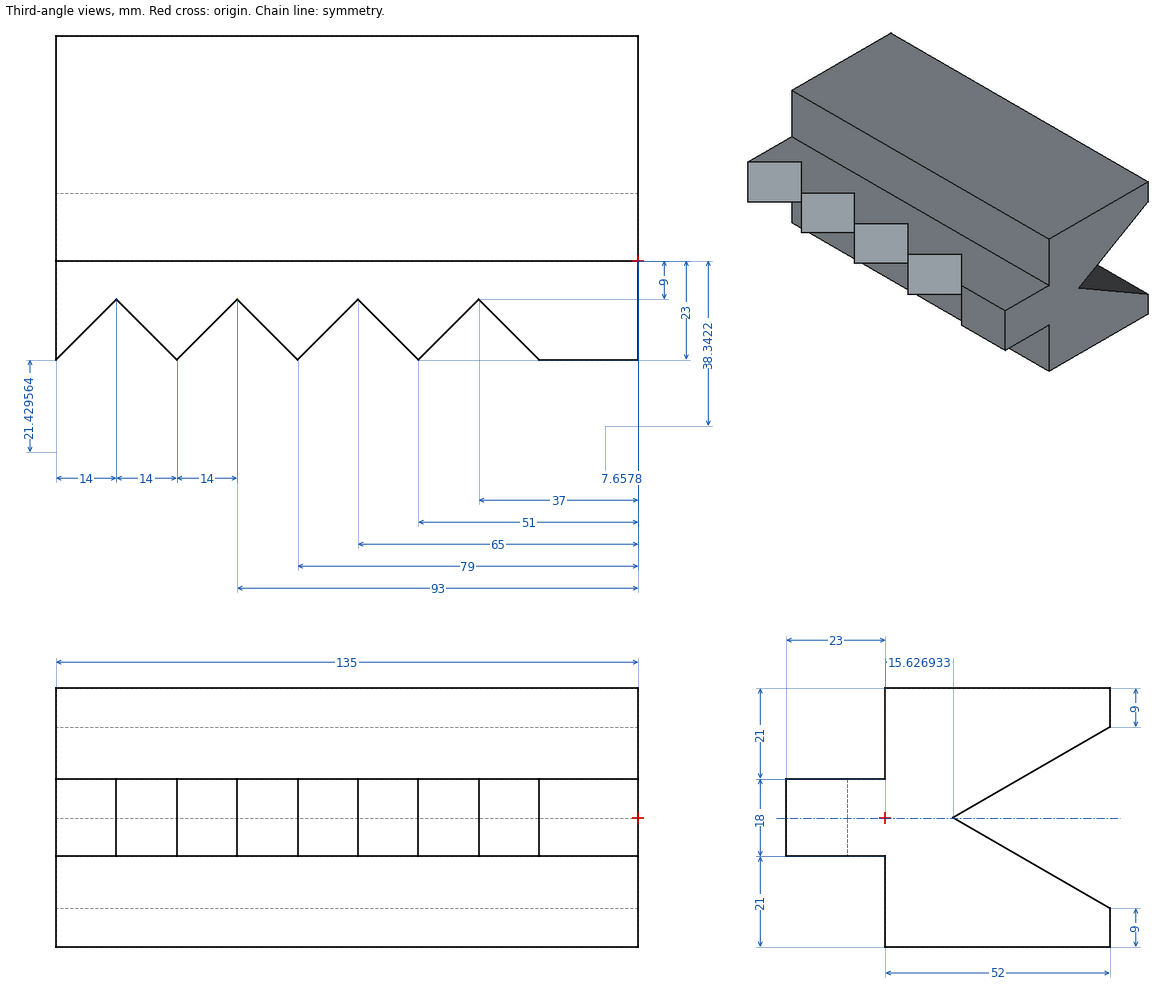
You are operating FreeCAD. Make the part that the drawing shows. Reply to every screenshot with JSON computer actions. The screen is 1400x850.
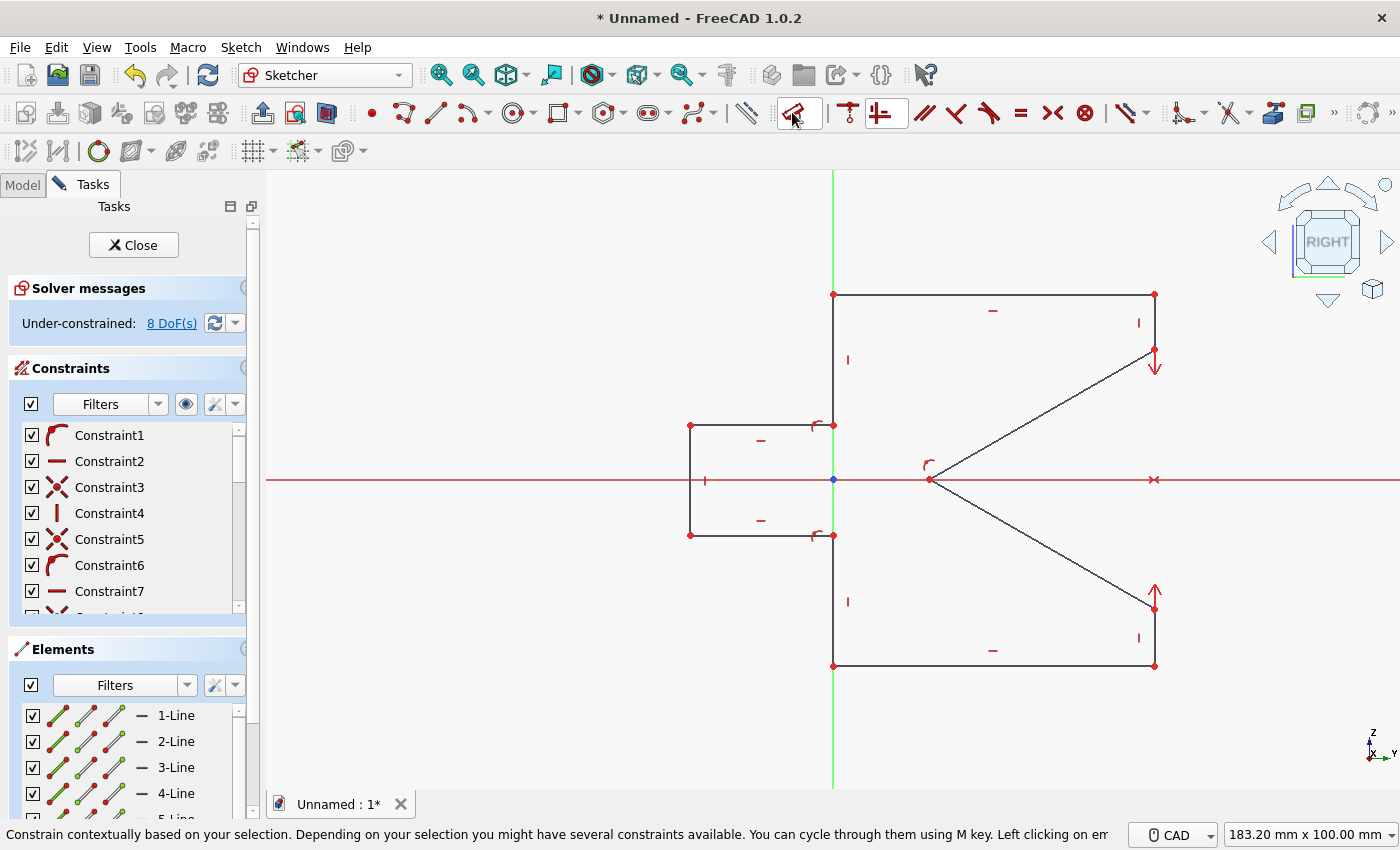
{"action": "left_click", "coordinate": [1155, 649]}
{"action": "left_click", "coordinate": [1189, 638]}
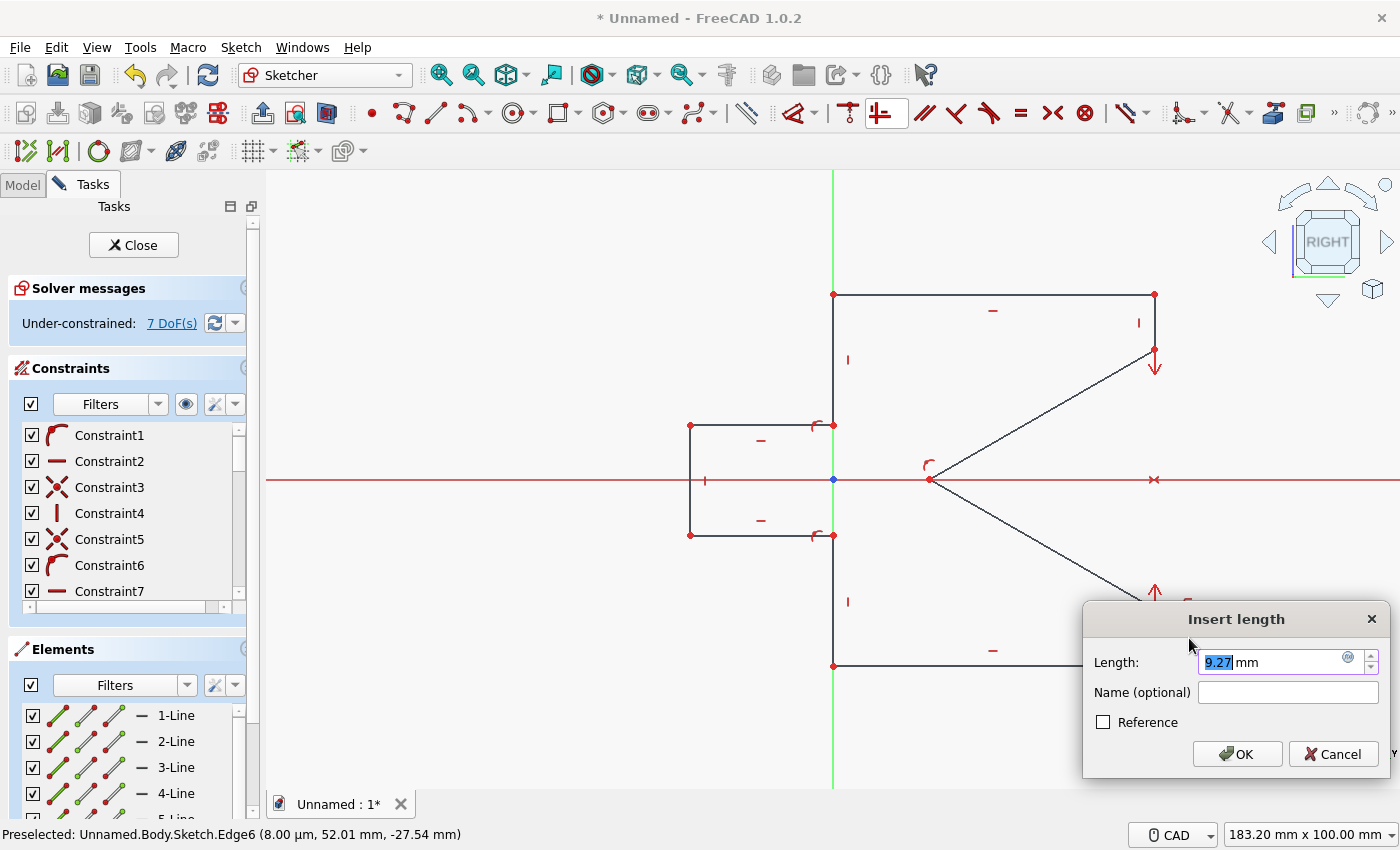
{"action": "type", "text": "9"}
{"action": "key", "text": "Return"}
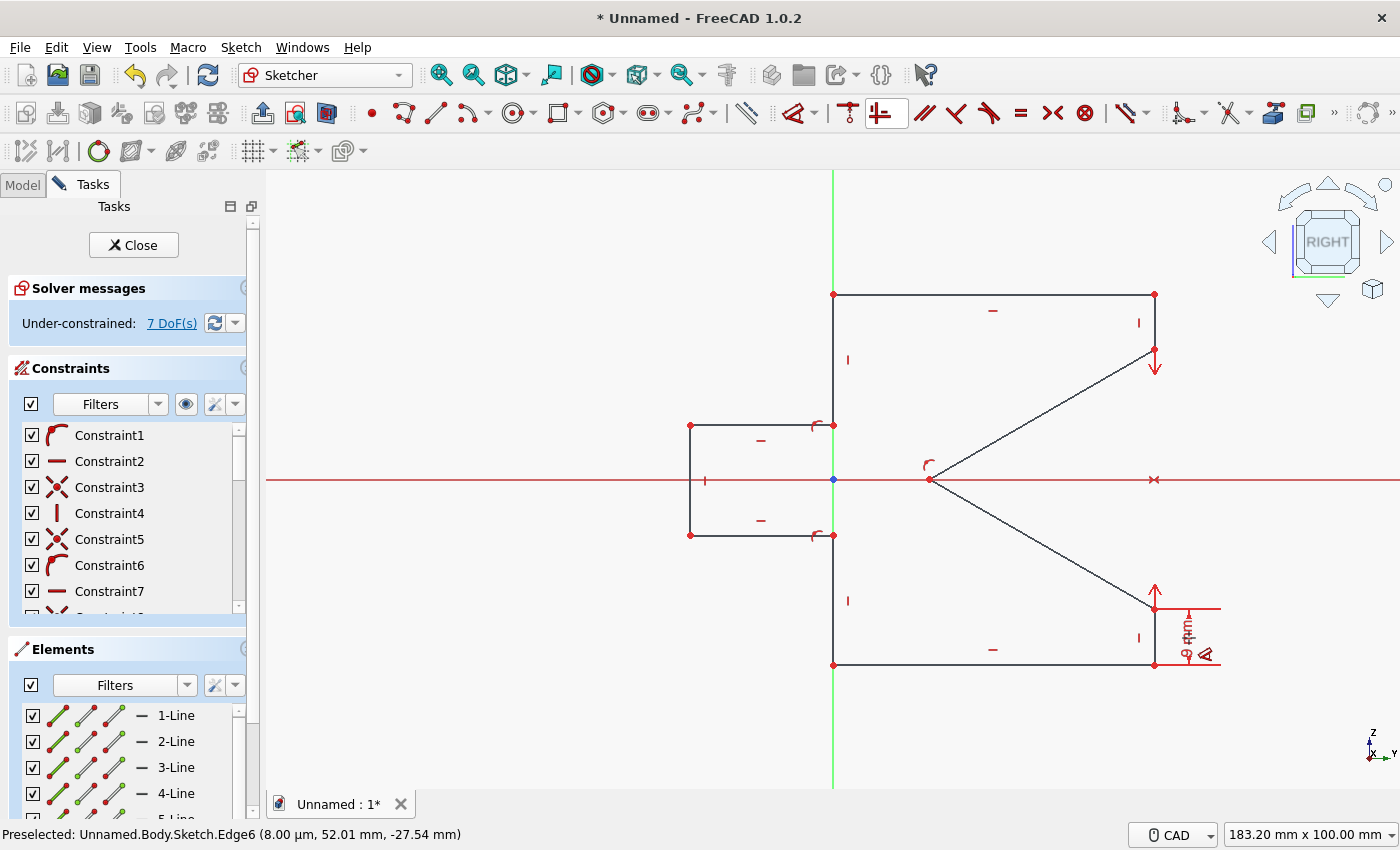
{"action": "left_click", "coordinate": [1155, 333]}
{"action": "left_click", "coordinate": [1189, 322]}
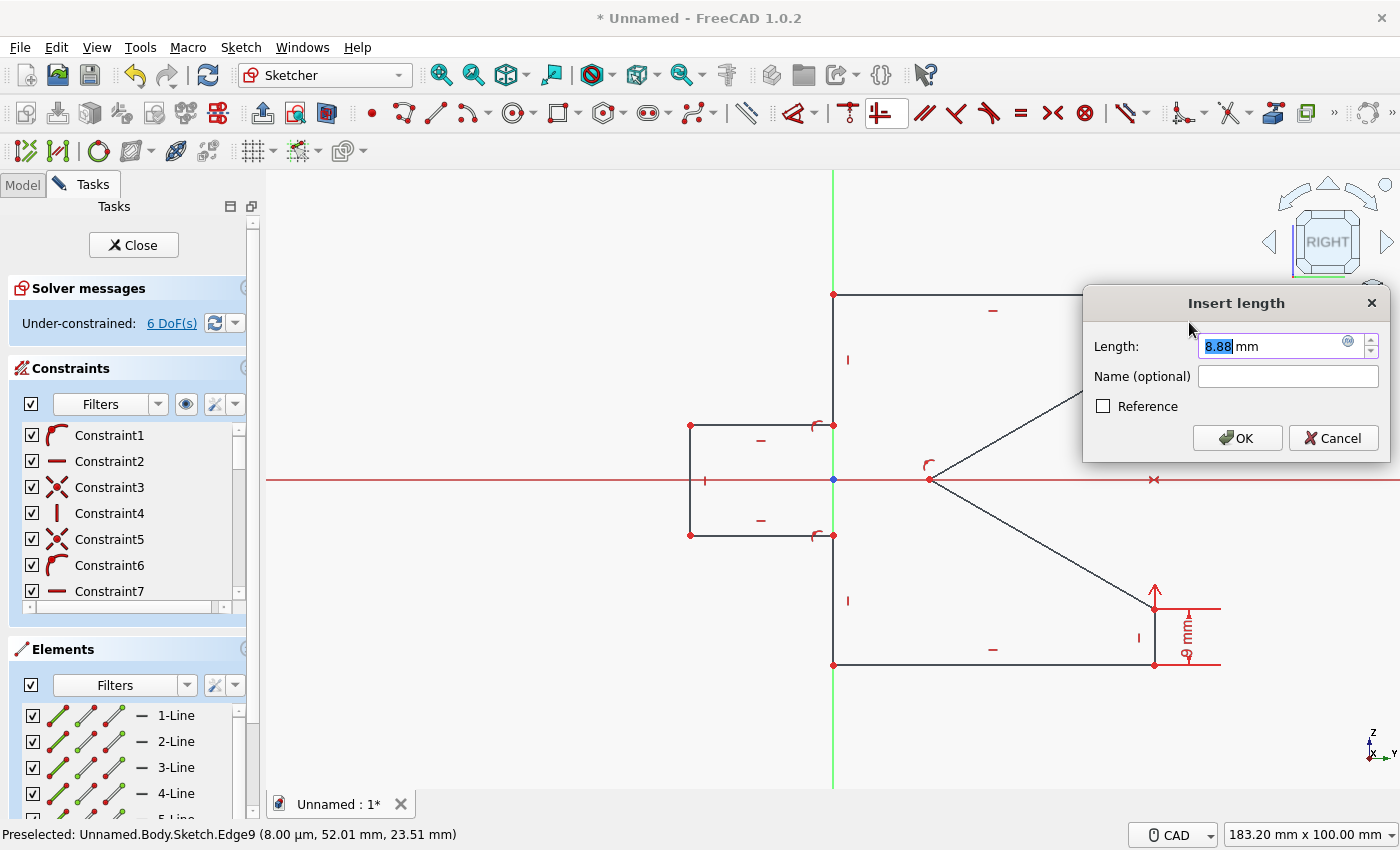
{"action": "type", "text": "9"}
{"action": "key", "text": "Return"}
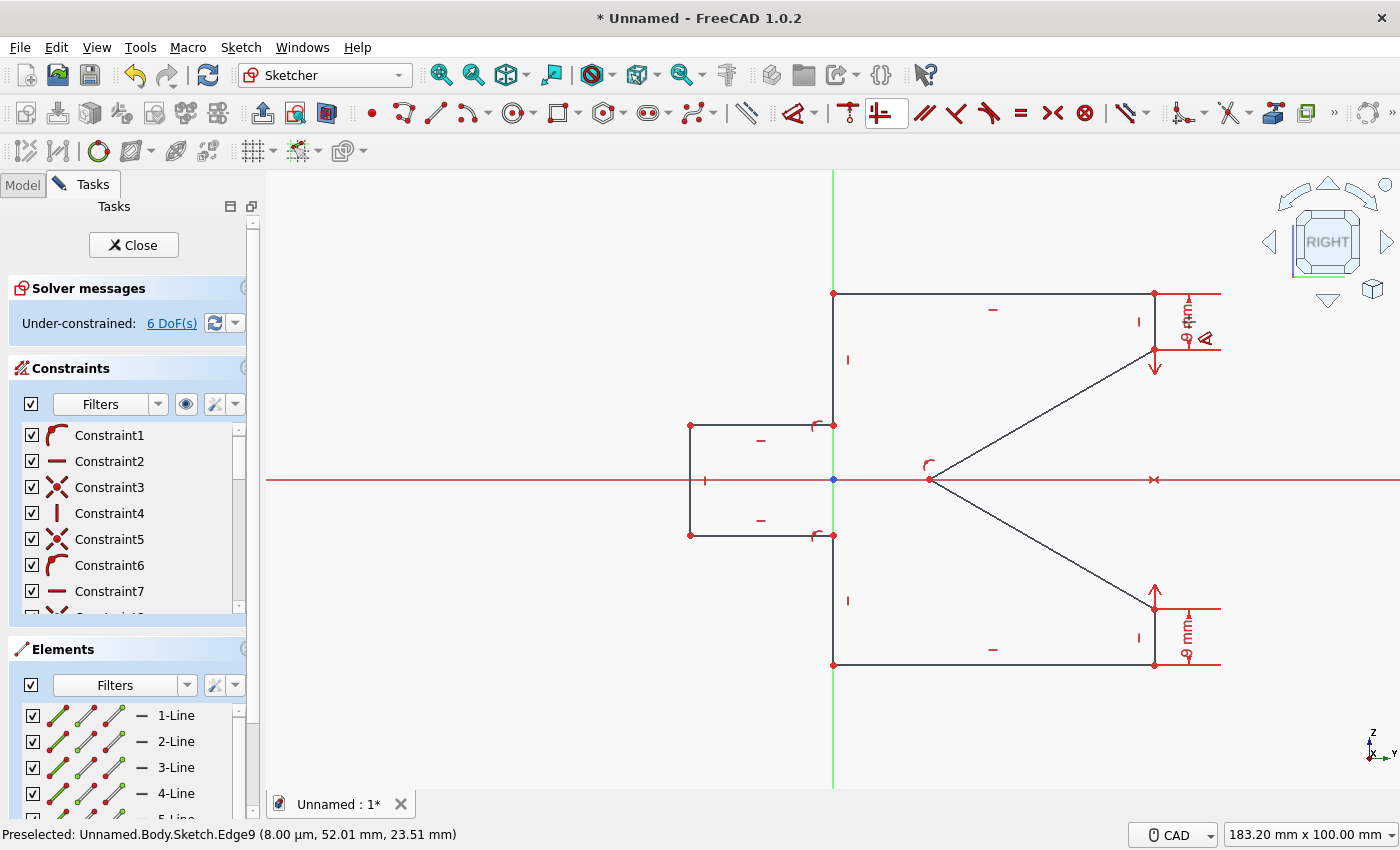
{"action": "left_click", "coordinate": [790, 425]}
{"action": "left_click", "coordinate": [762, 391]}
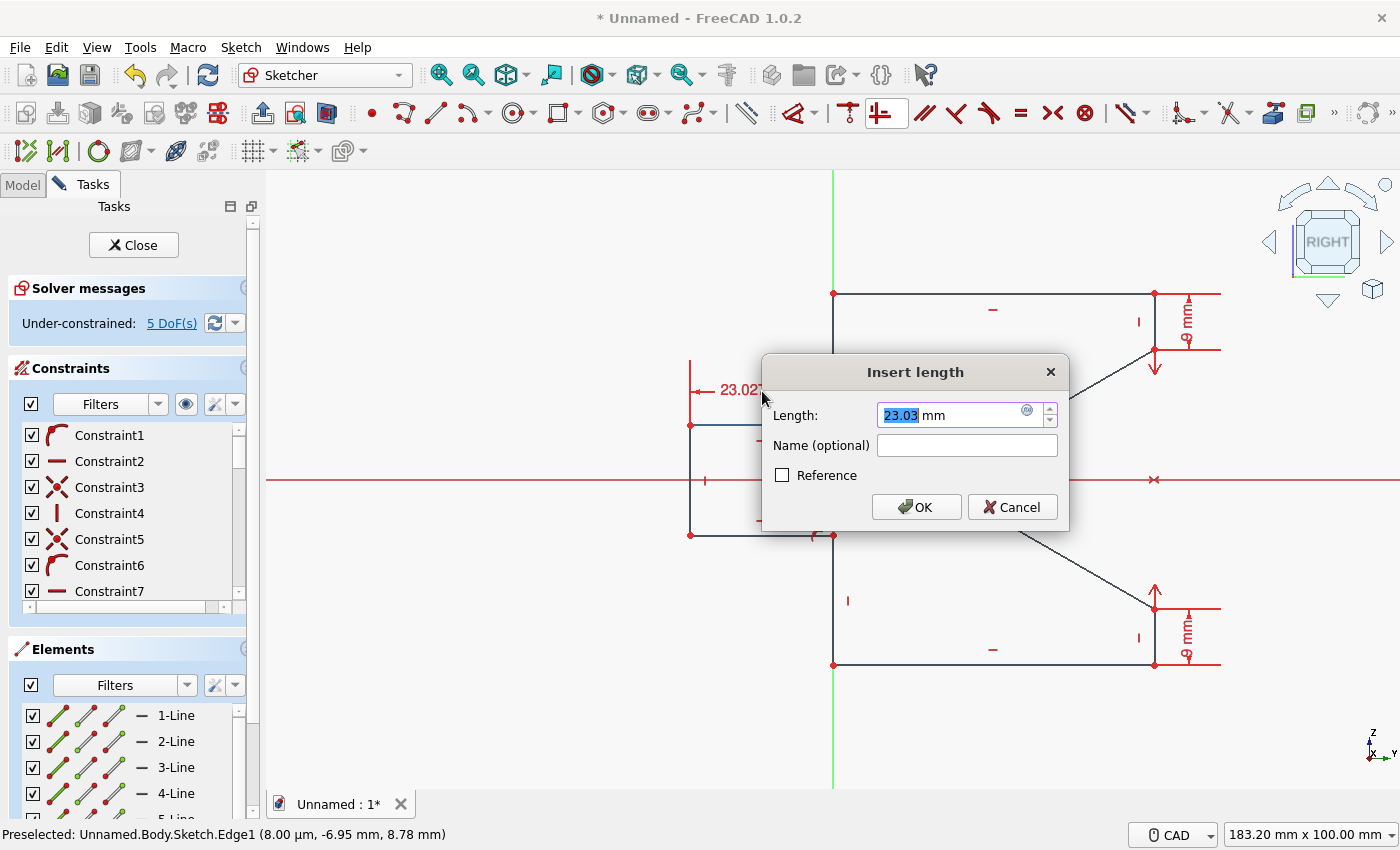
{"action": "type", "text": "23"}
{"action": "key", "text": "Return"}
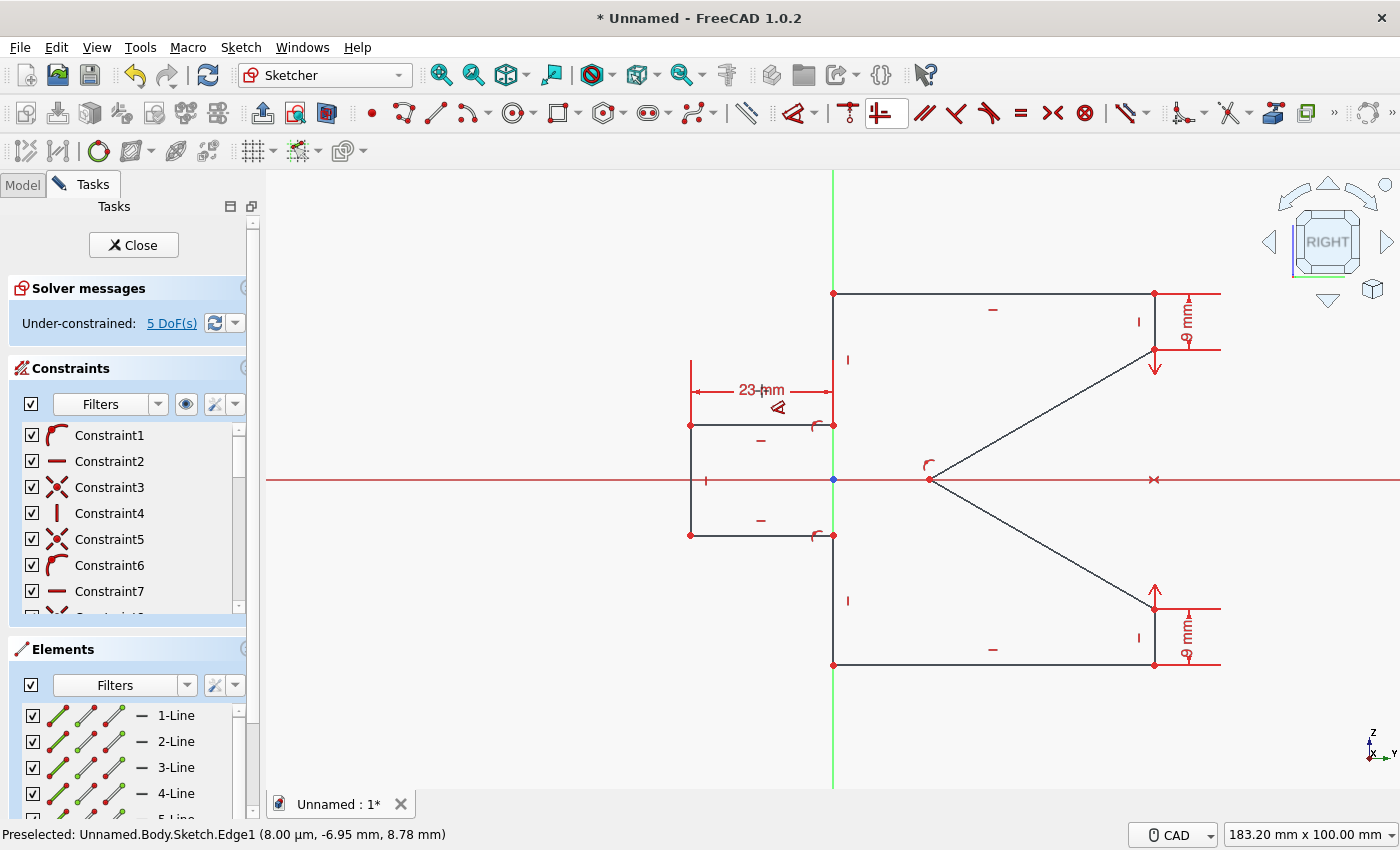
{"action": "left_click", "coordinate": [691, 458]}
{"action": "left_click", "coordinate": [657, 455]}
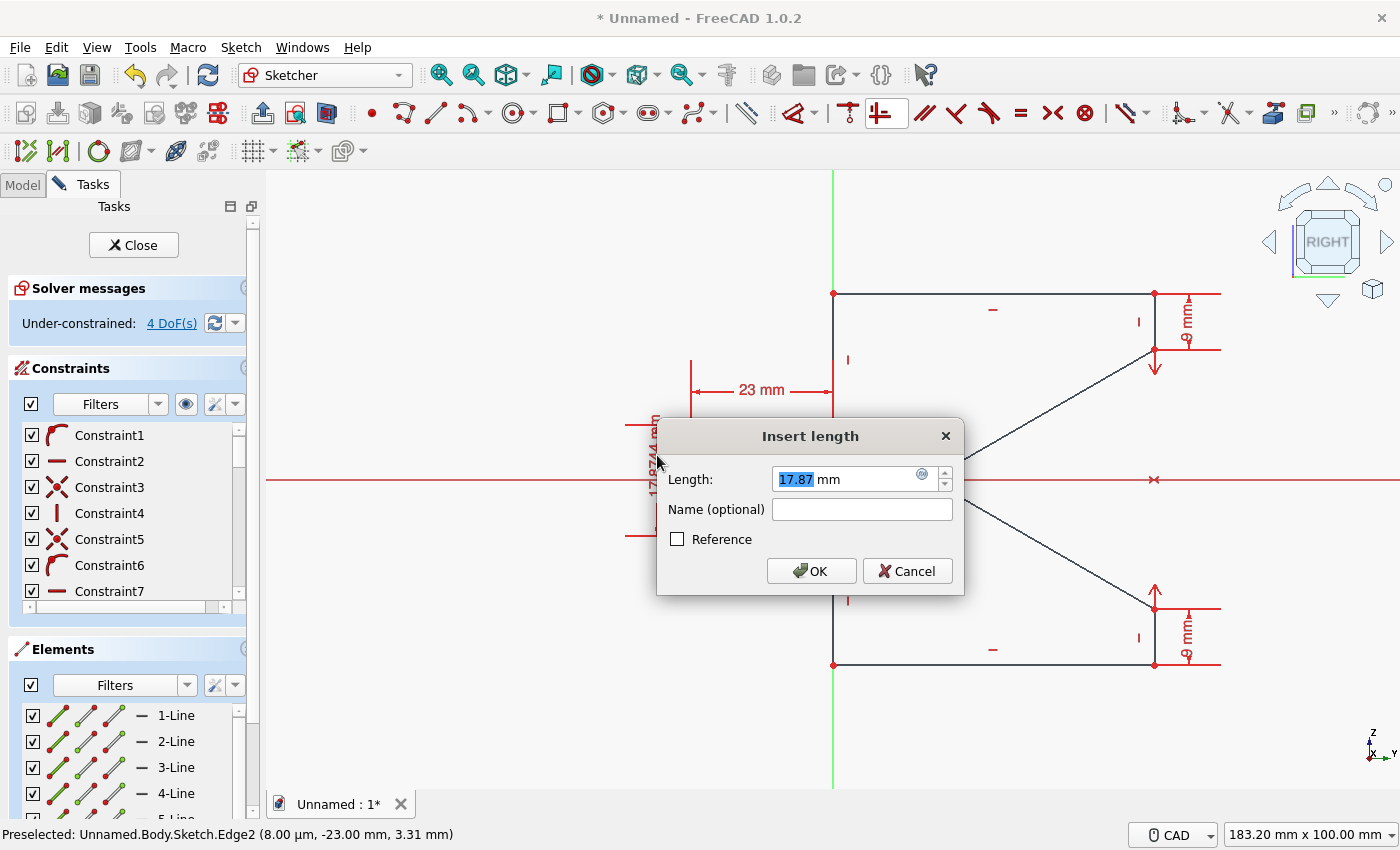
{"action": "type", "text": "18"}
{"action": "key", "text": "Return"}